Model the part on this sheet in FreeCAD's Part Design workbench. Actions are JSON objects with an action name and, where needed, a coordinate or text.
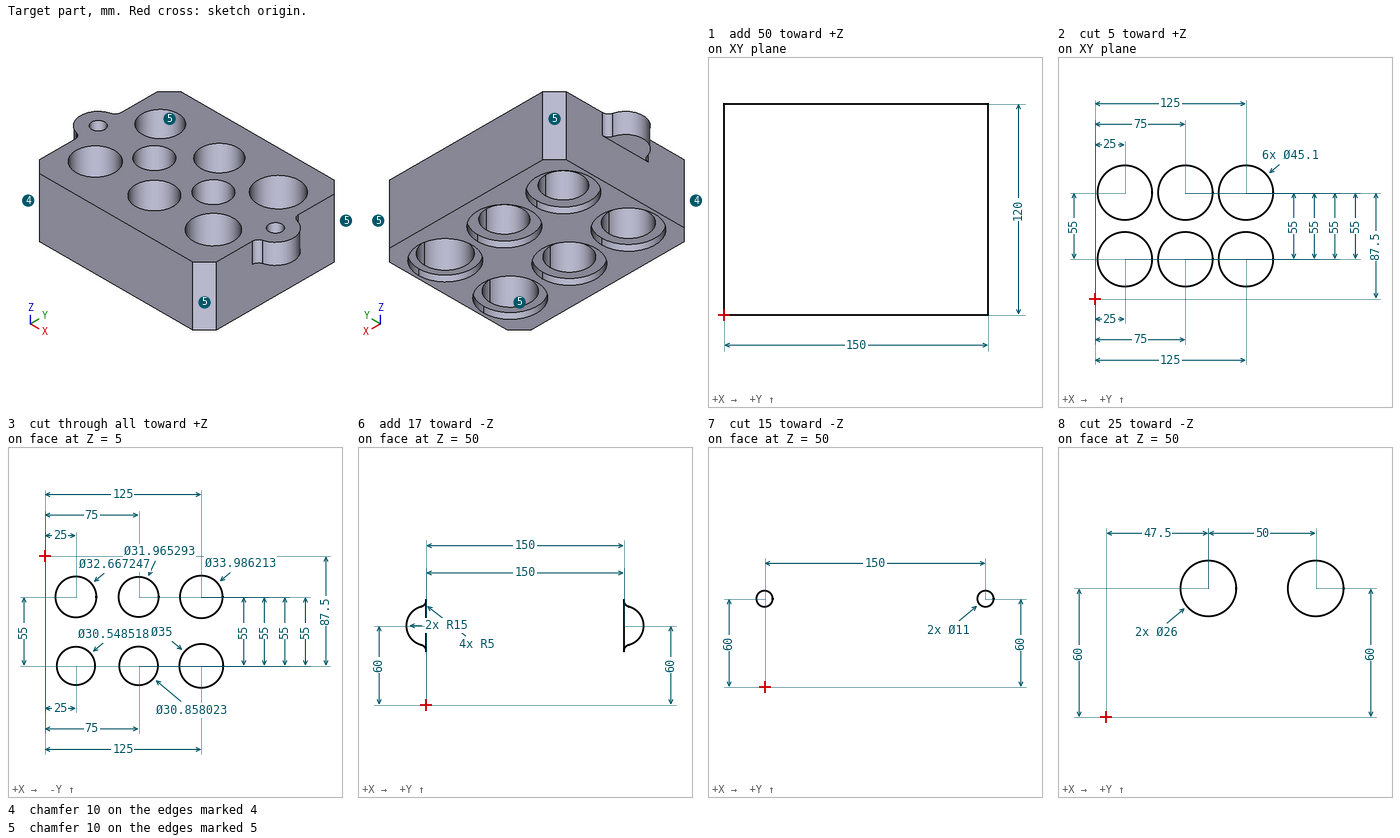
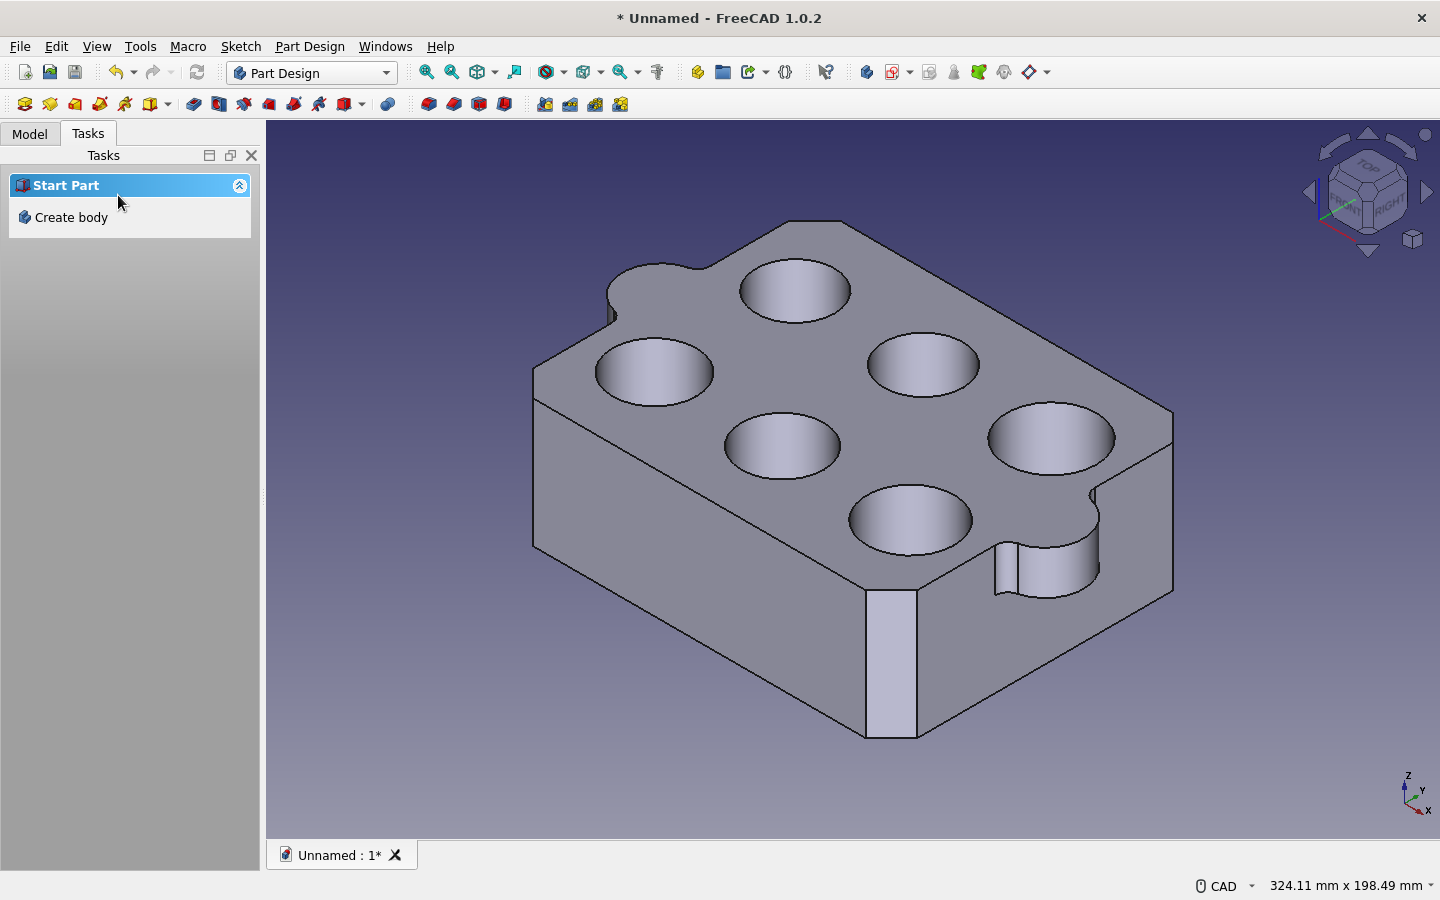
{"action": "left_click", "coordinate": [787, 367]}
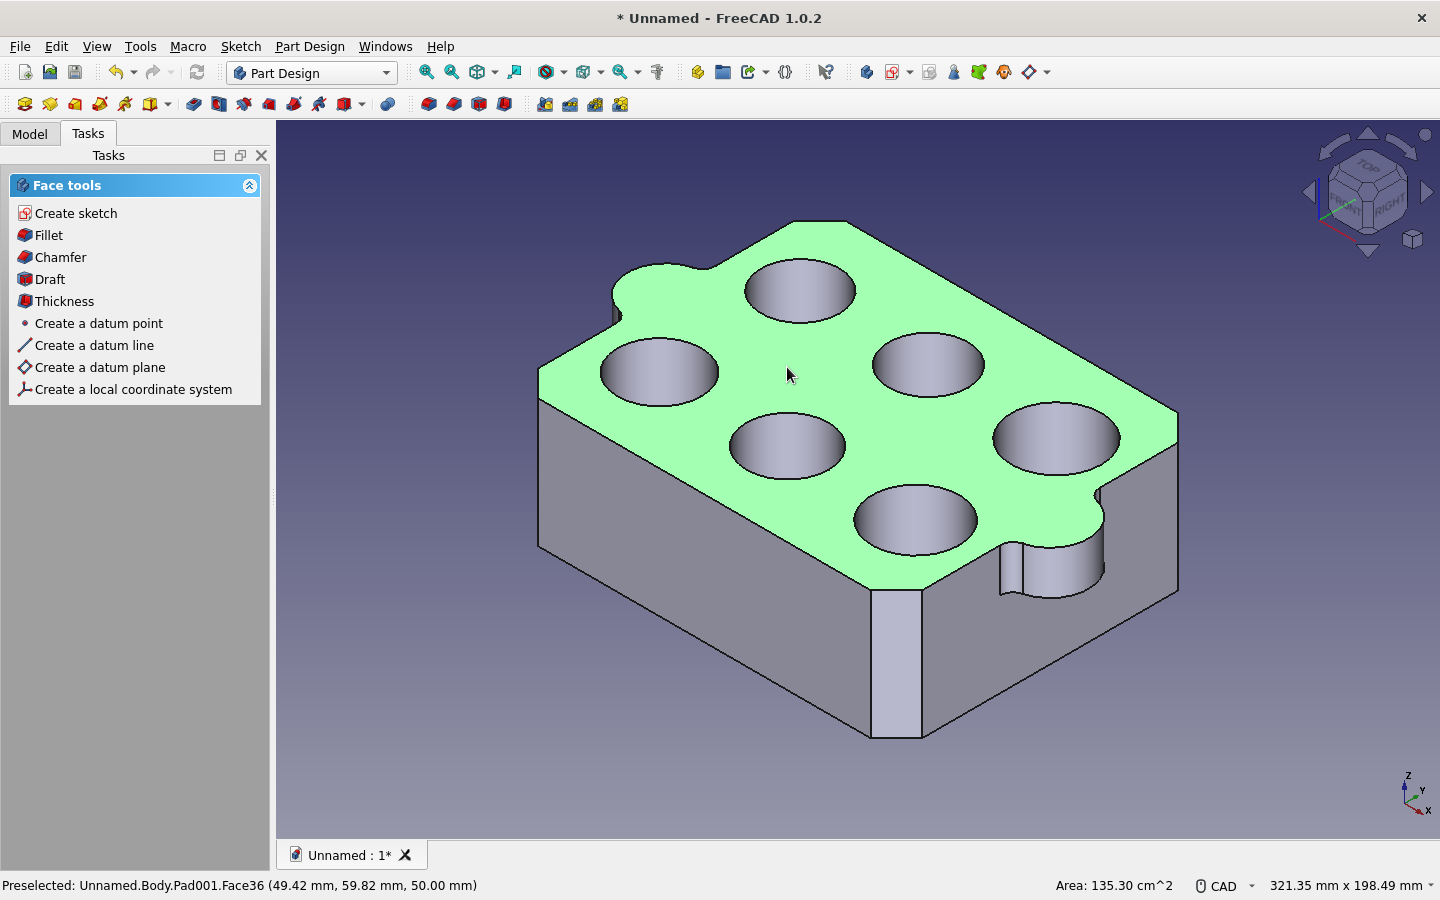
{"action": "left_click", "coordinate": [892, 72]}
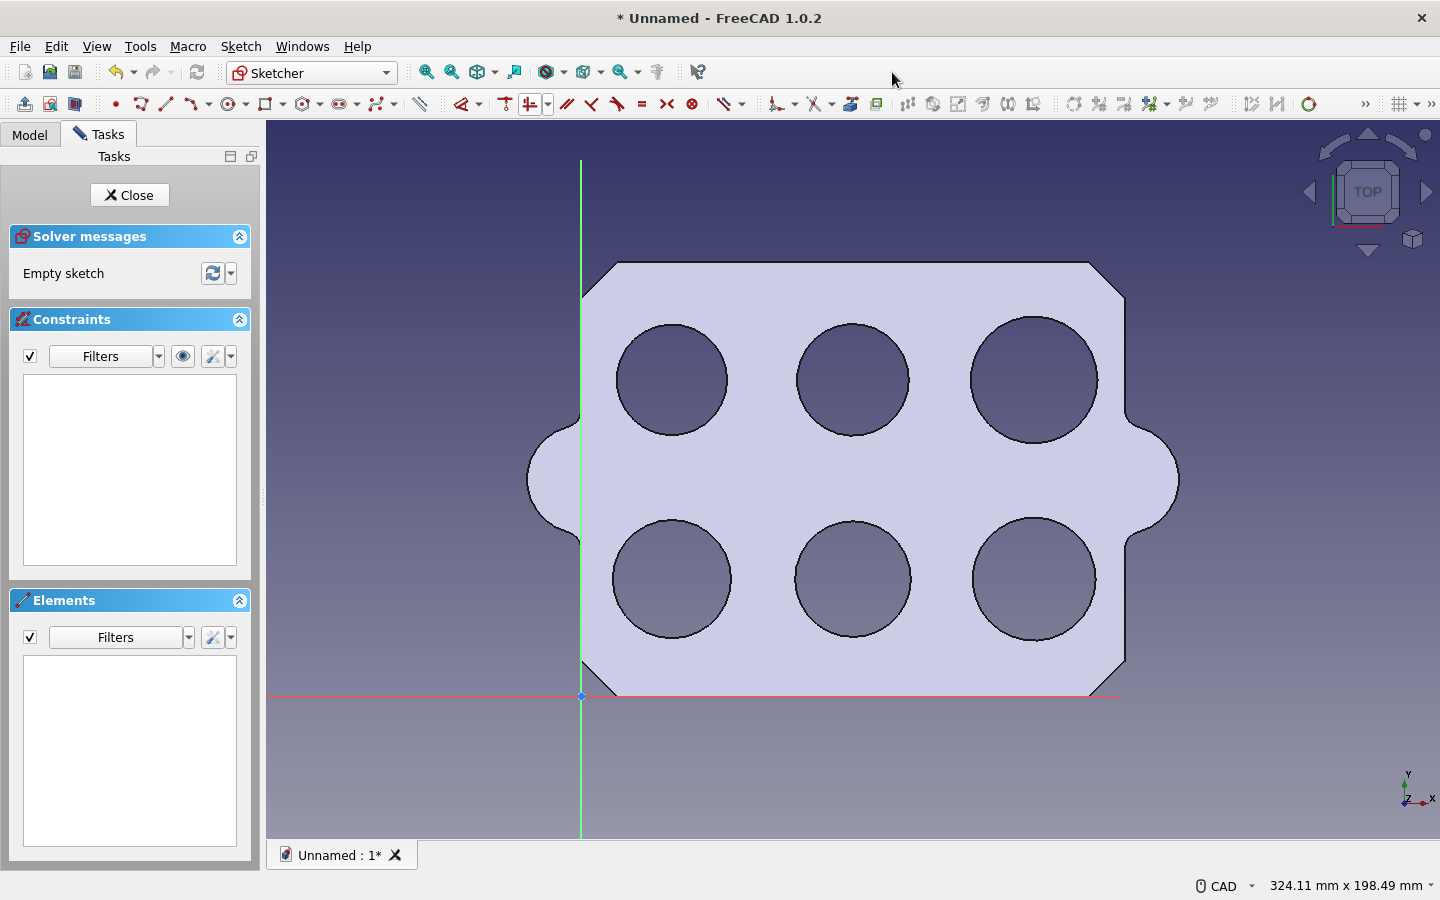
{"action": "left_click", "coordinate": [228, 104]}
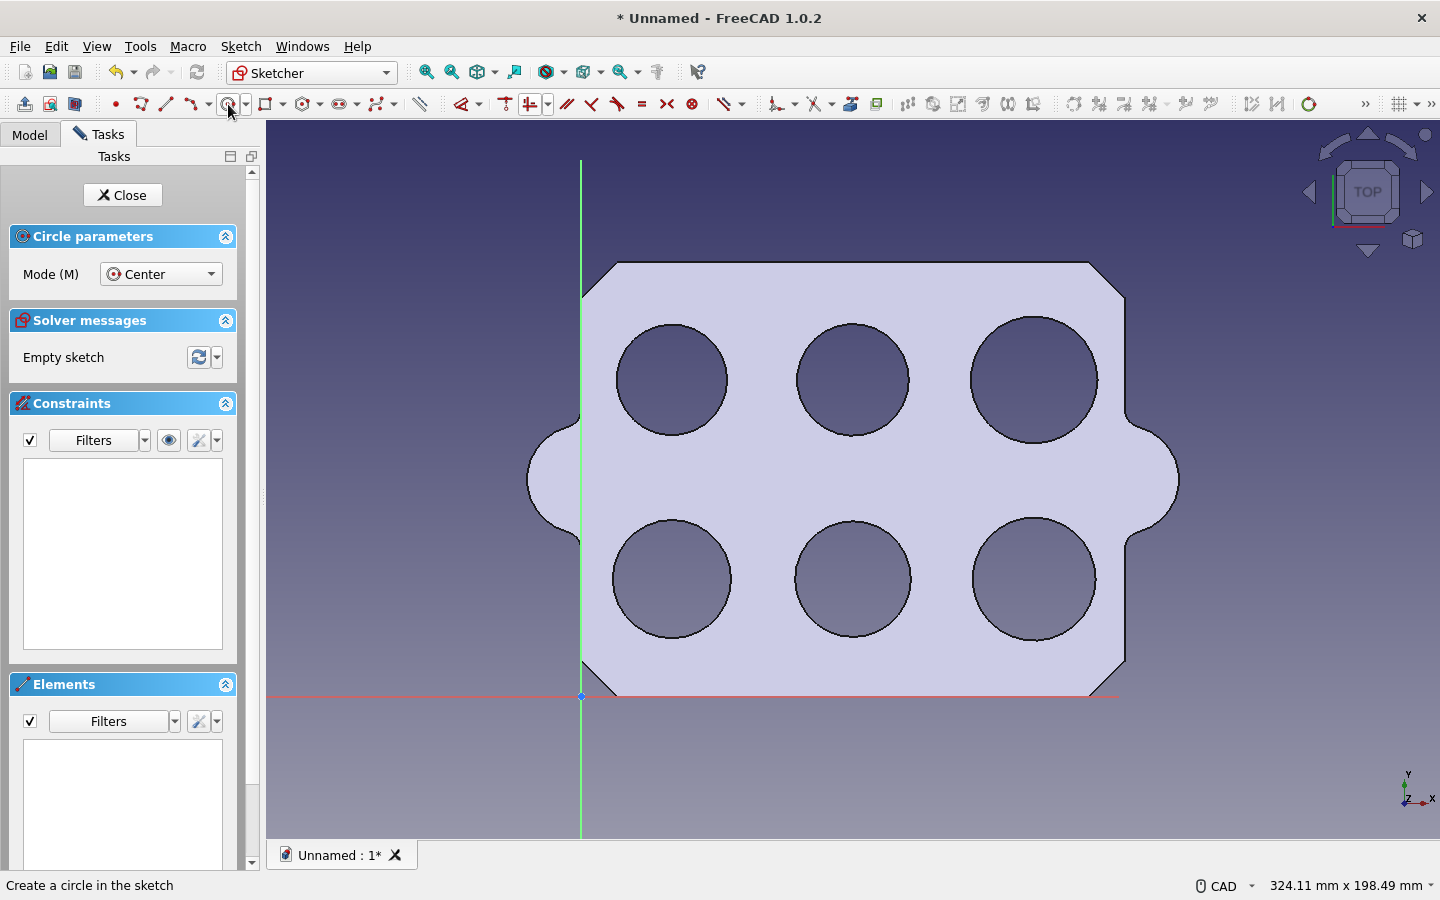
{"action": "left_click", "coordinate": [1125, 480]}
{"action": "left_click", "coordinate": [1139, 465]}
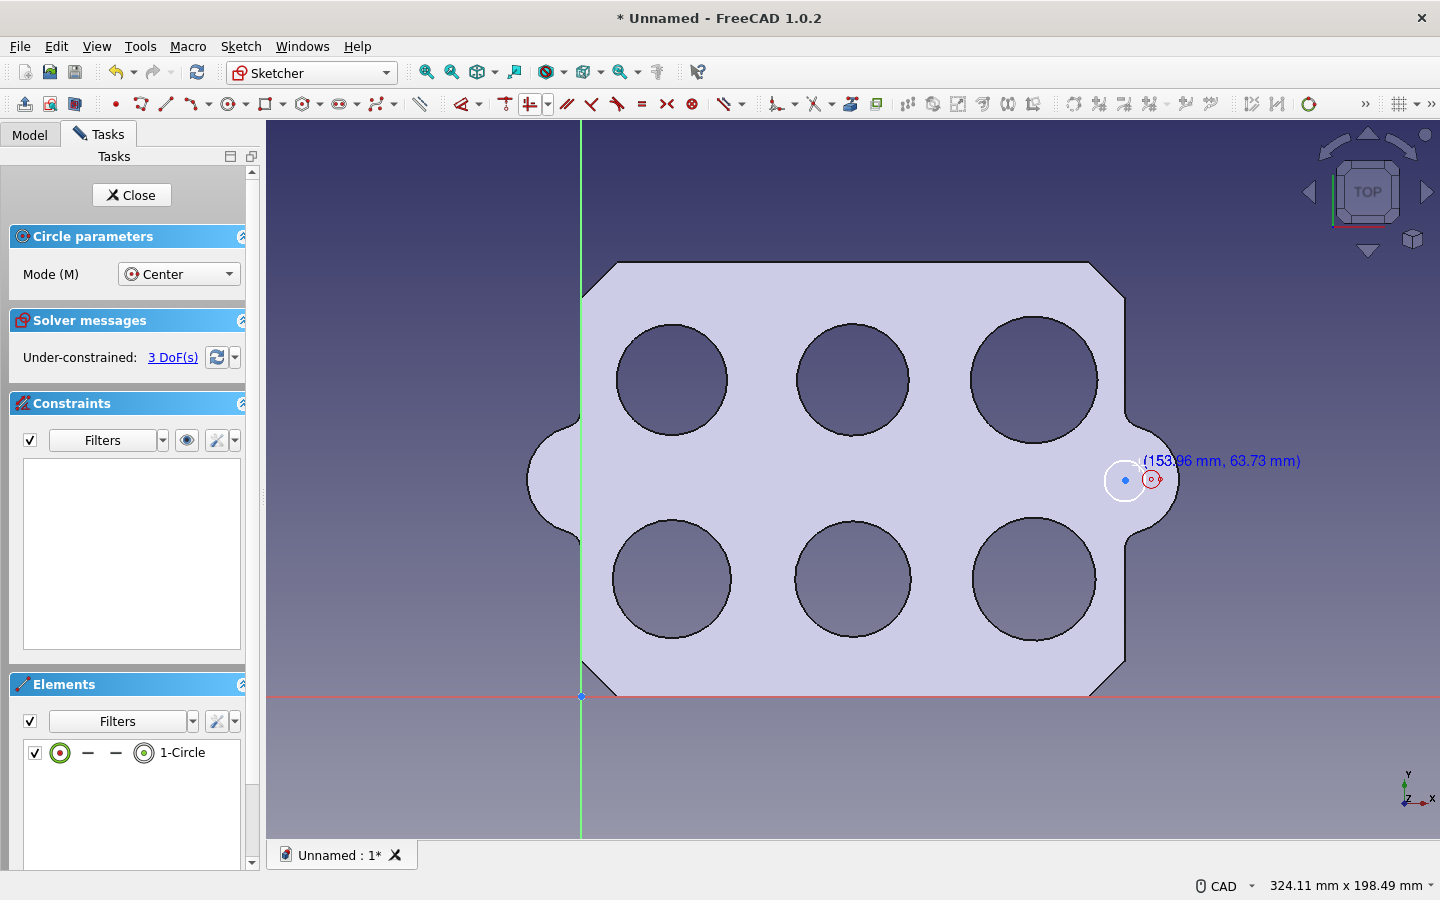
{"action": "left_click", "coordinate": [581, 480]}
{"action": "left_click", "coordinate": [595, 465]}
{"action": "key", "text": "Escape"}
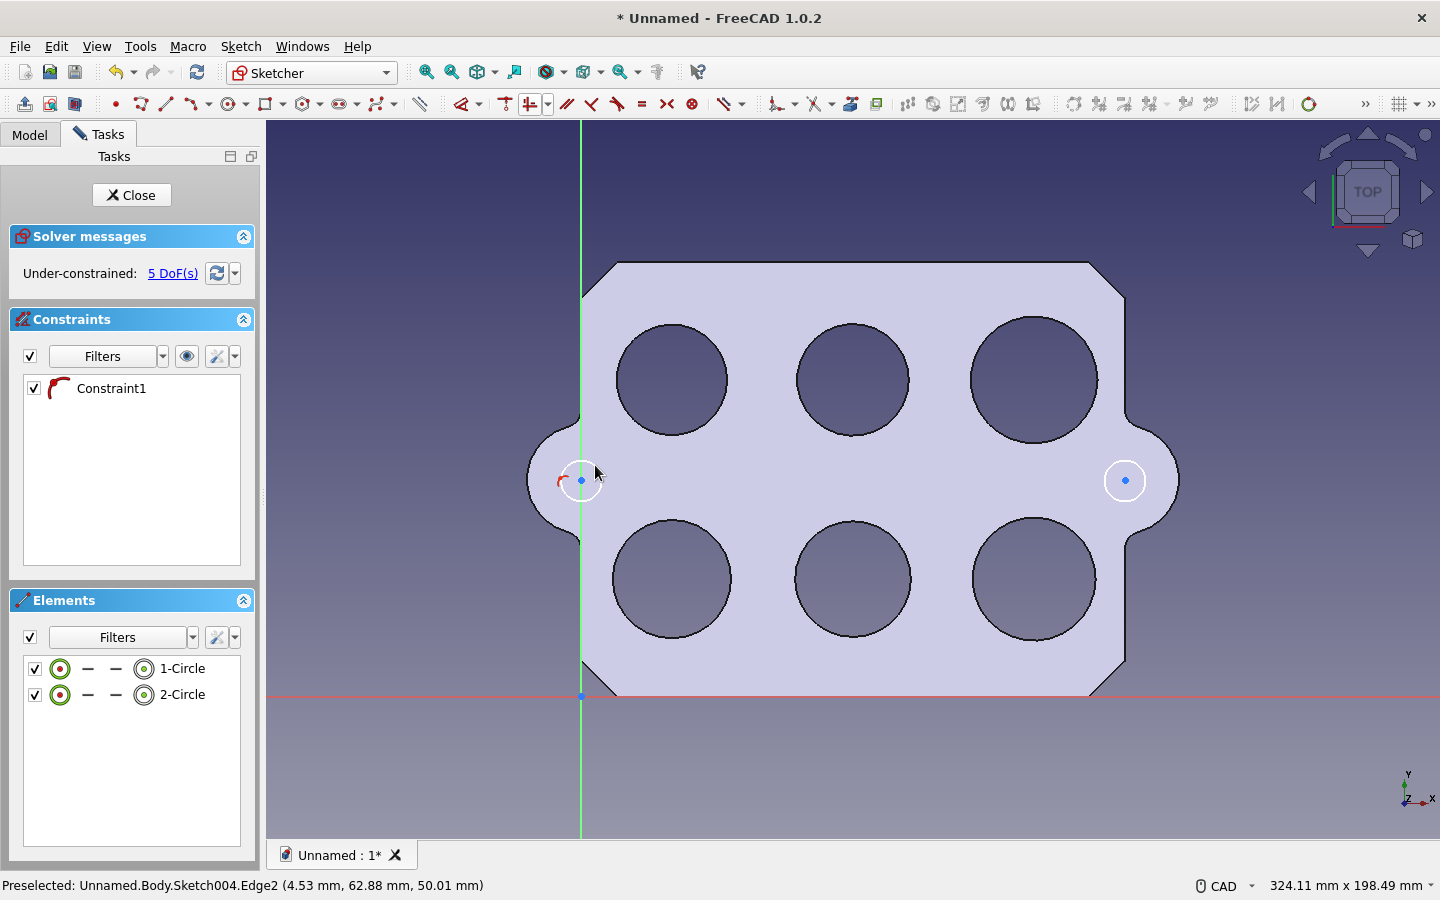
{"action": "left_click", "coordinate": [1139, 466]}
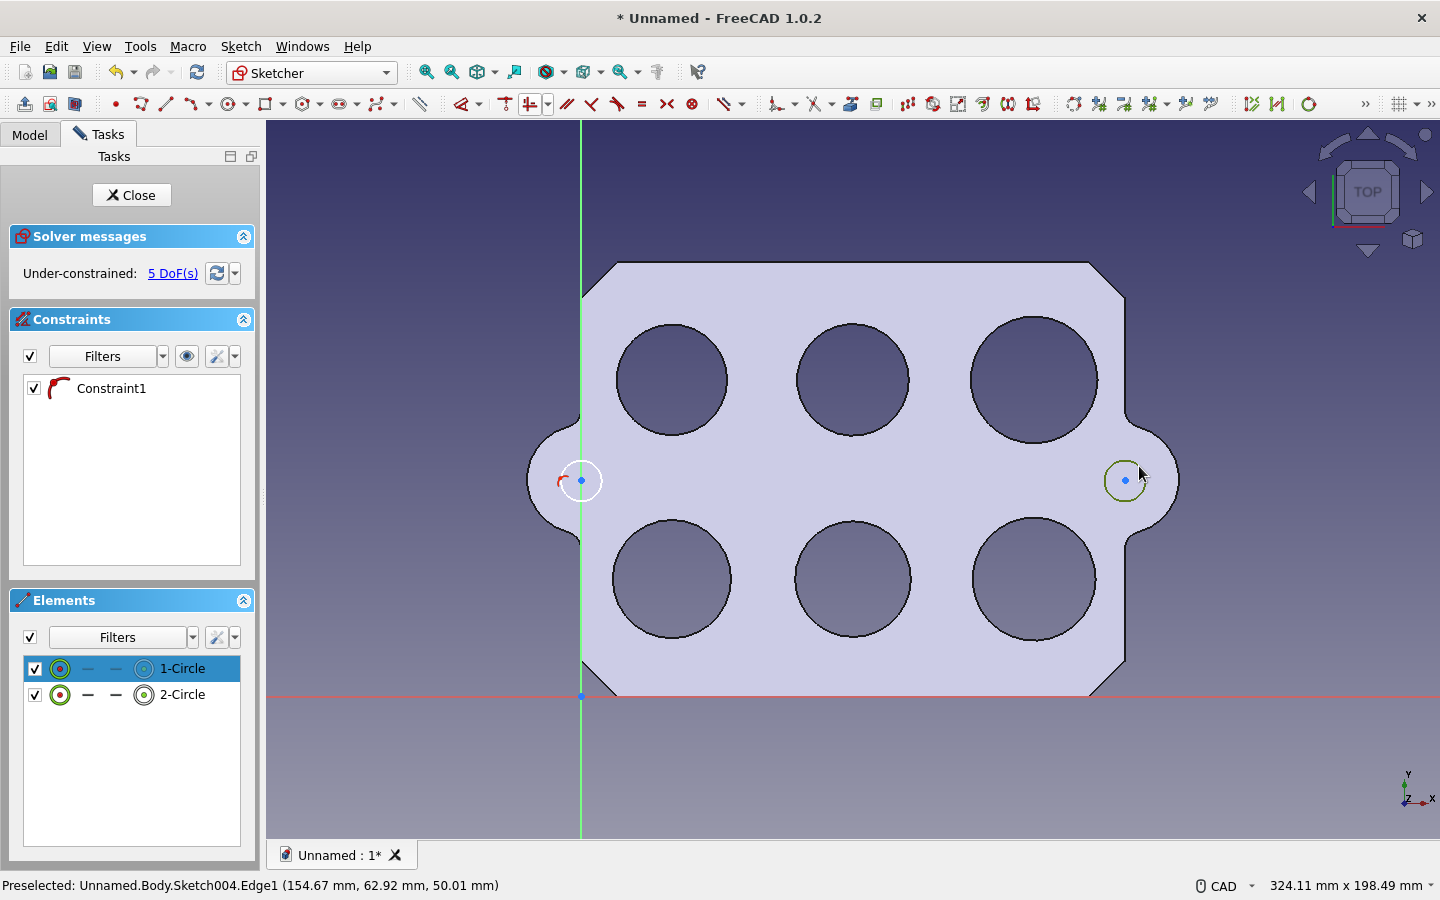
{"action": "left_click", "coordinate": [596, 467]}